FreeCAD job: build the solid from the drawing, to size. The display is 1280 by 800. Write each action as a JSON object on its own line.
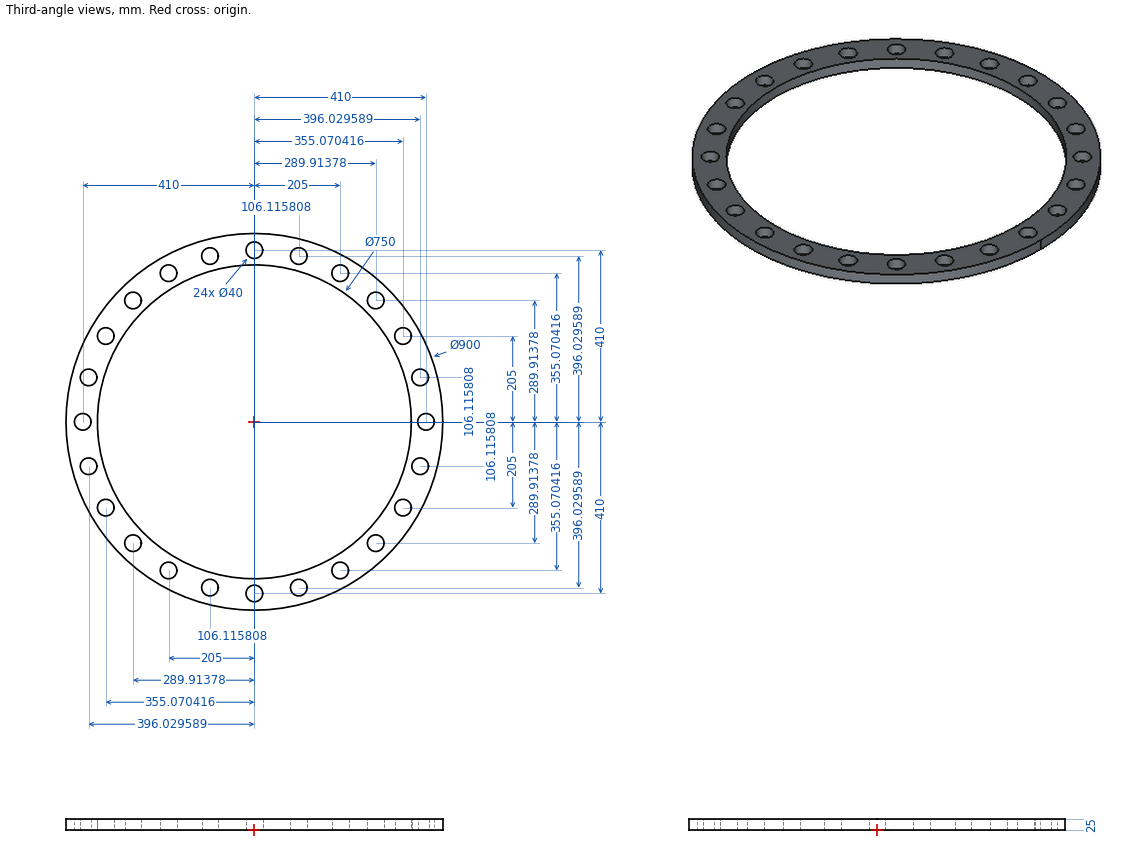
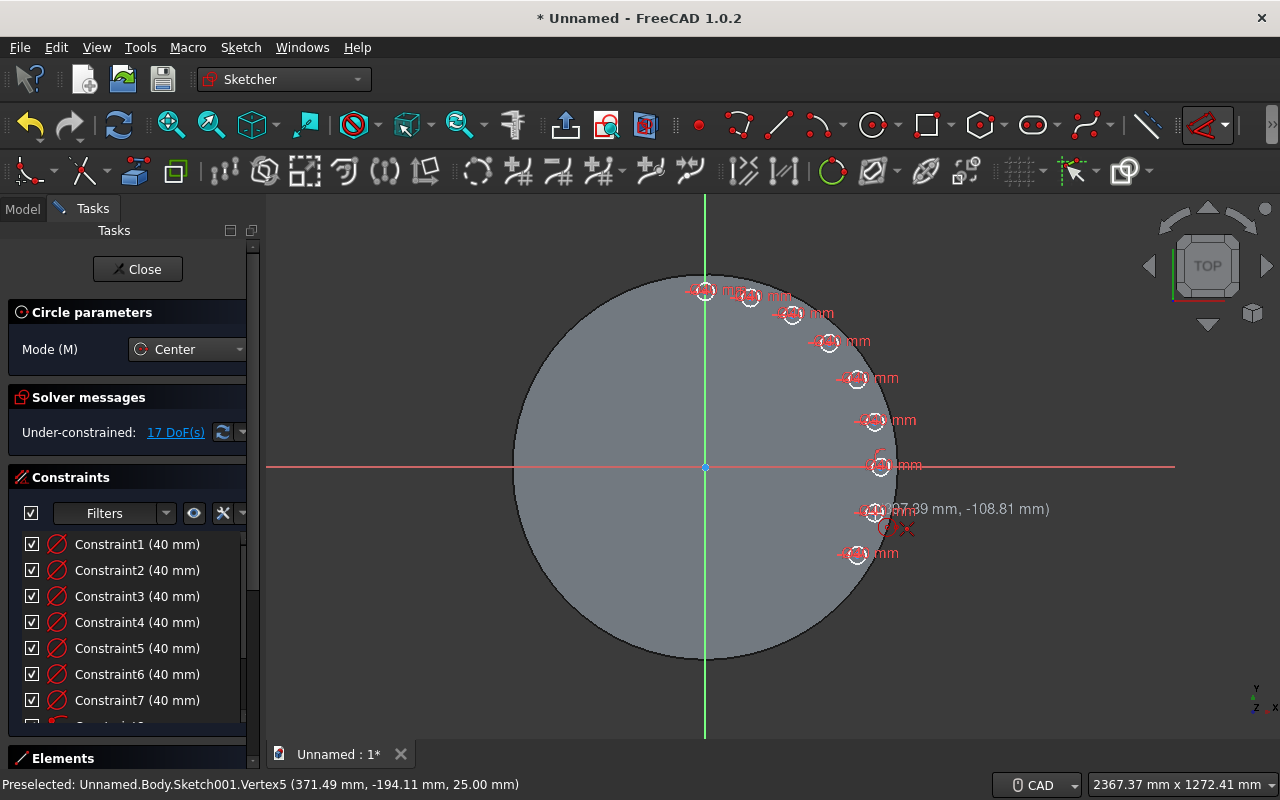
{"action": "scroll", "coordinate": [829, 591], "scroll_direction": "up", "scroll_amount": 5}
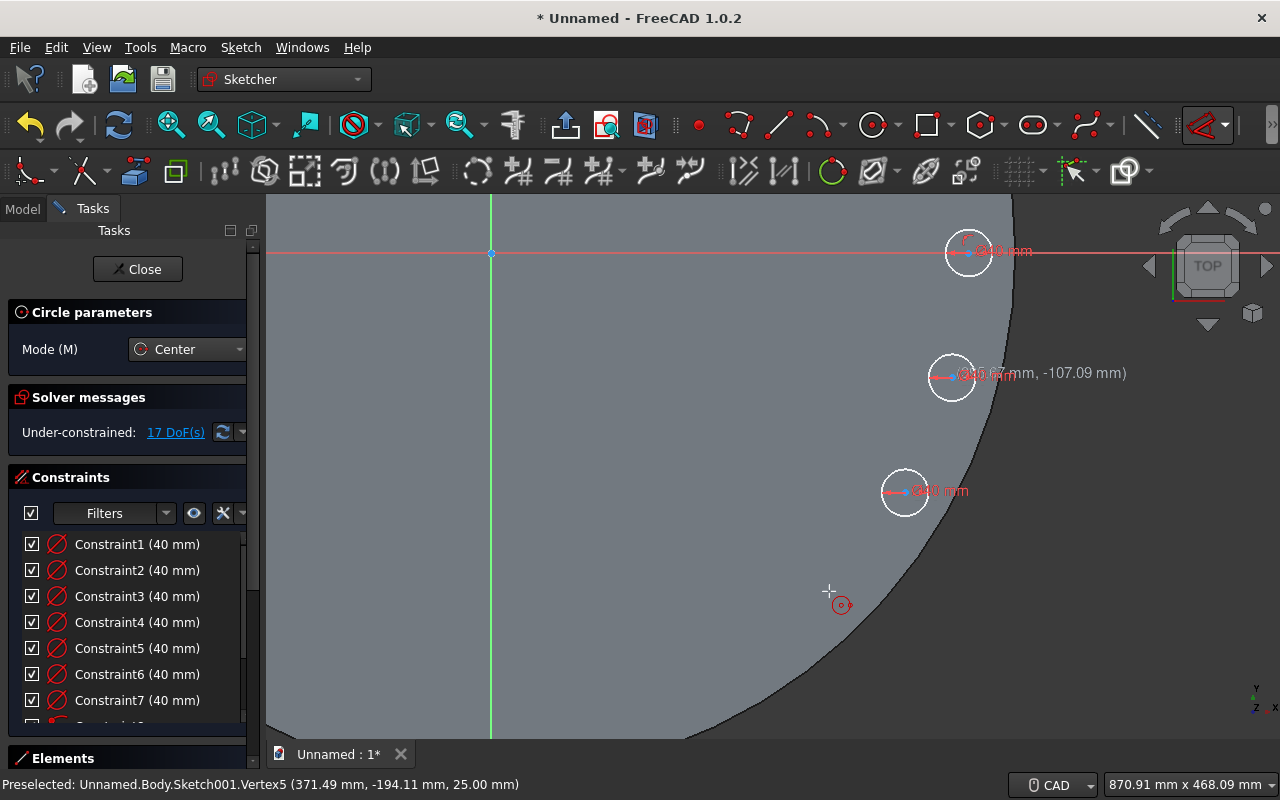
{"action": "left_click", "coordinate": [829, 591]}
{"action": "mouse_move", "coordinate": [845, 574]}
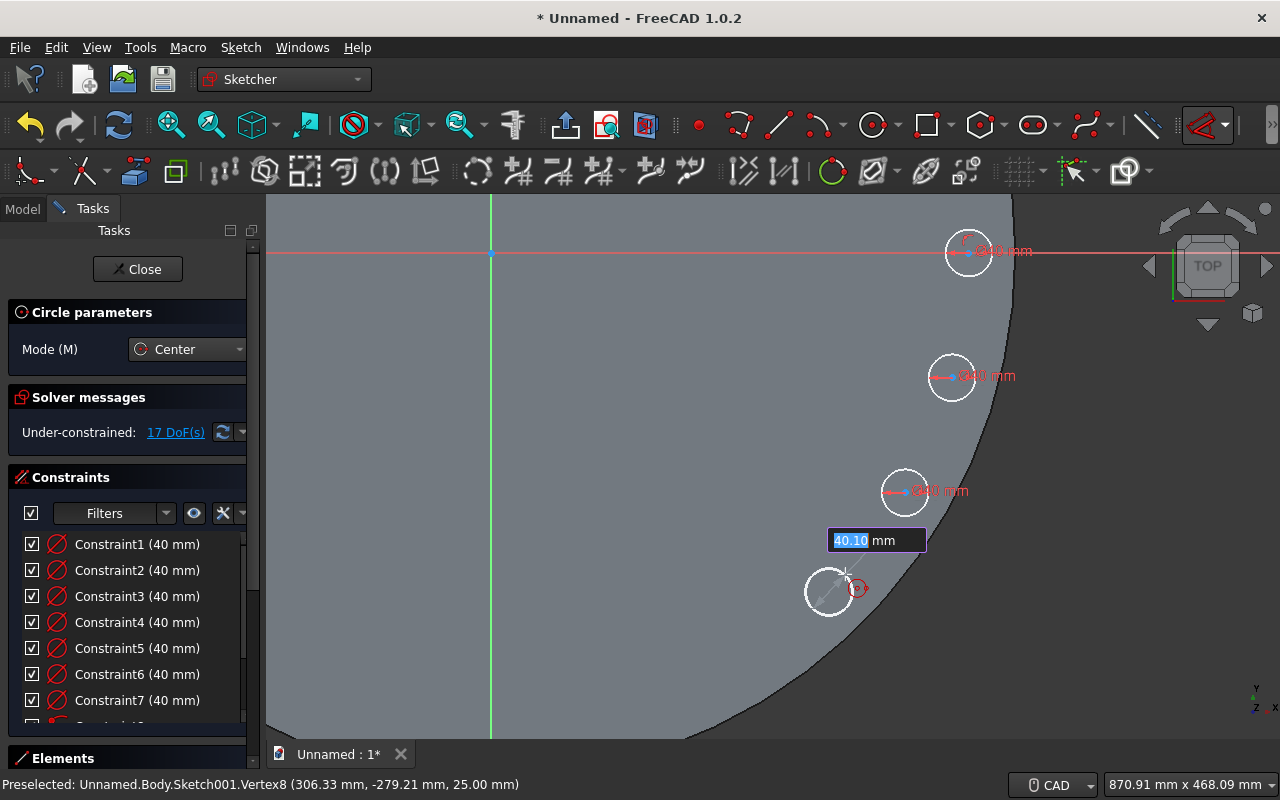
{"action": "type", "text": "40"}
{"action": "key", "text": "Return"}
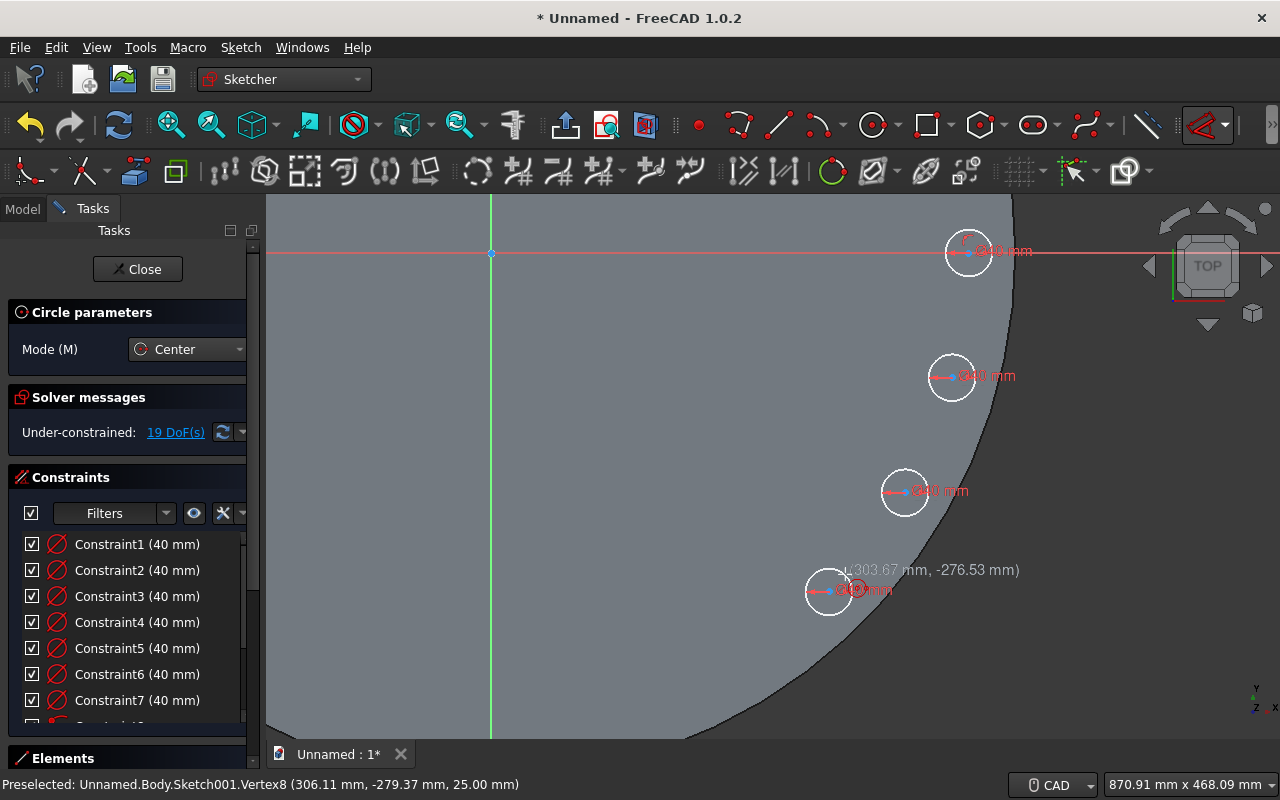
{"action": "left_click", "coordinate": [730, 666]}
{"action": "mouse_move", "coordinate": [747, 650]}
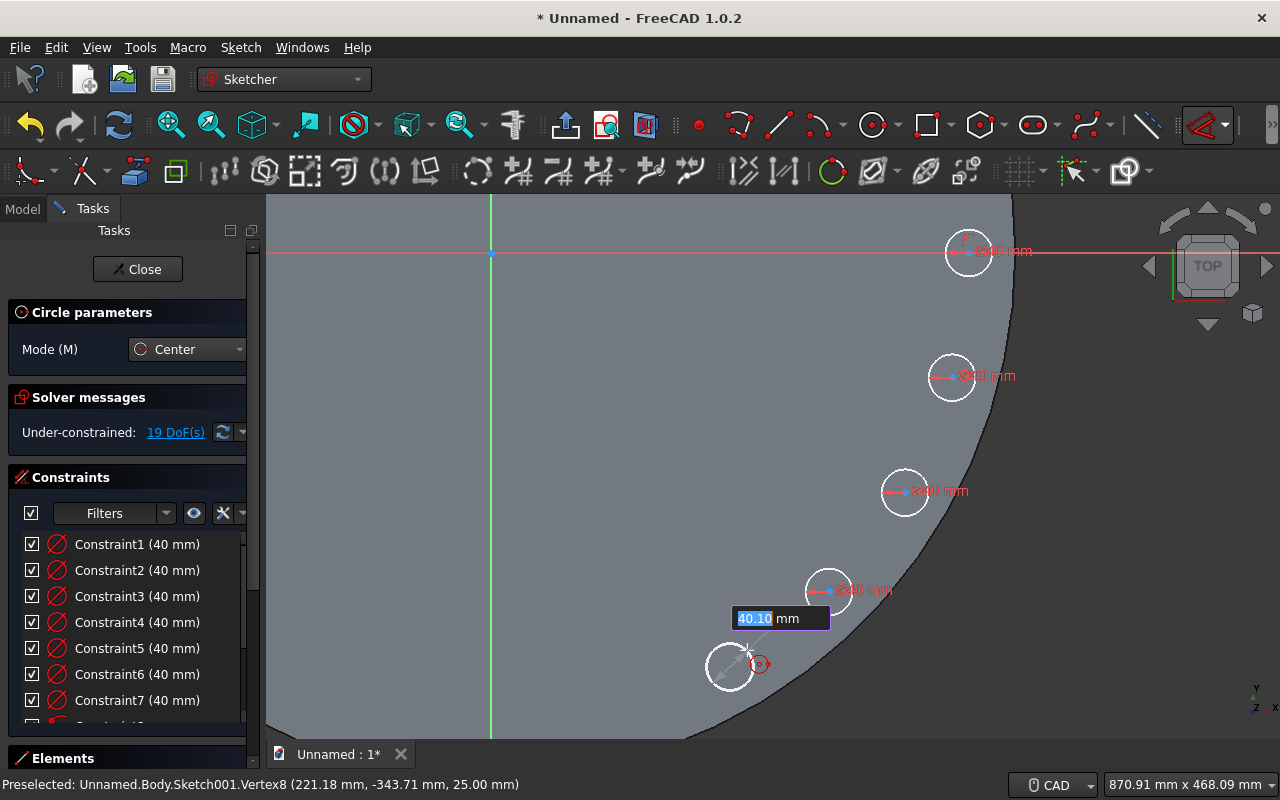
{"action": "type", "text": "40"}
{"action": "key", "text": "Return"}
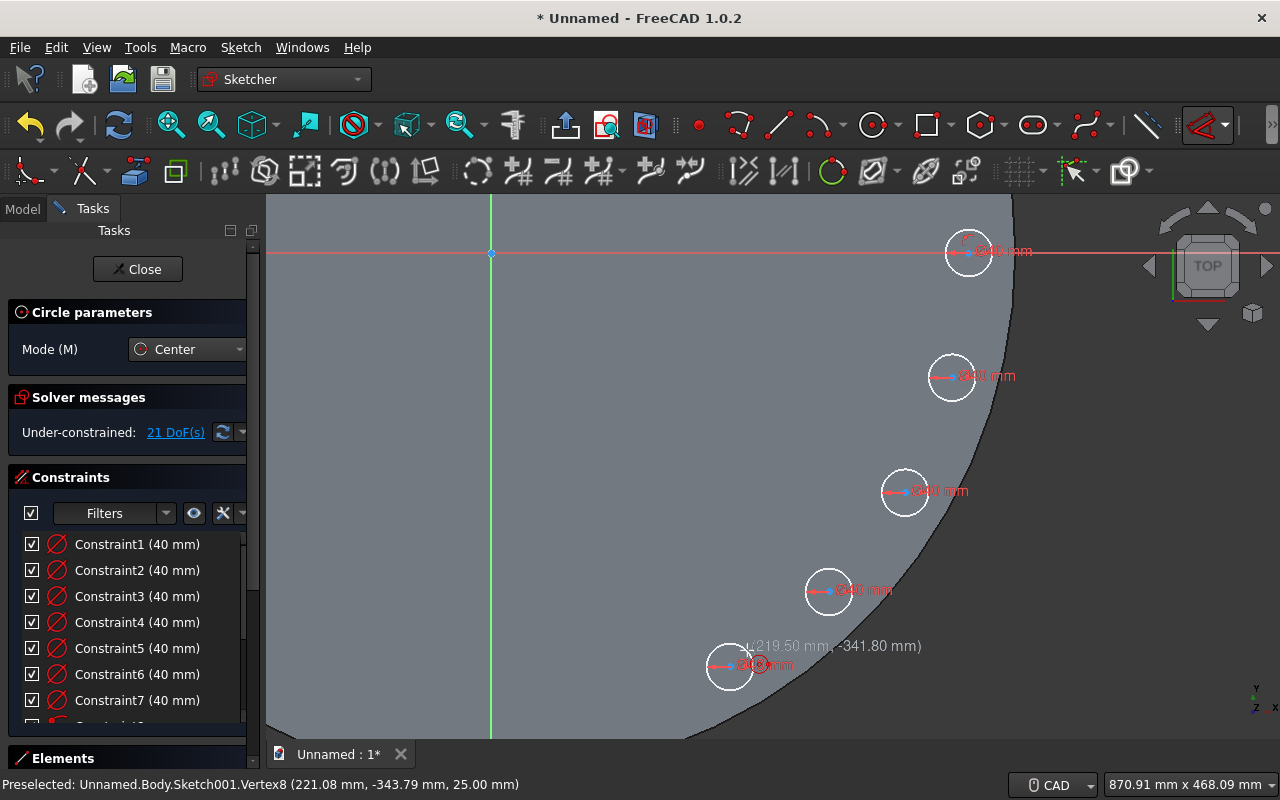
{"action": "scroll", "coordinate": [828, 591], "scroll_direction": "down", "scroll_amount": 5}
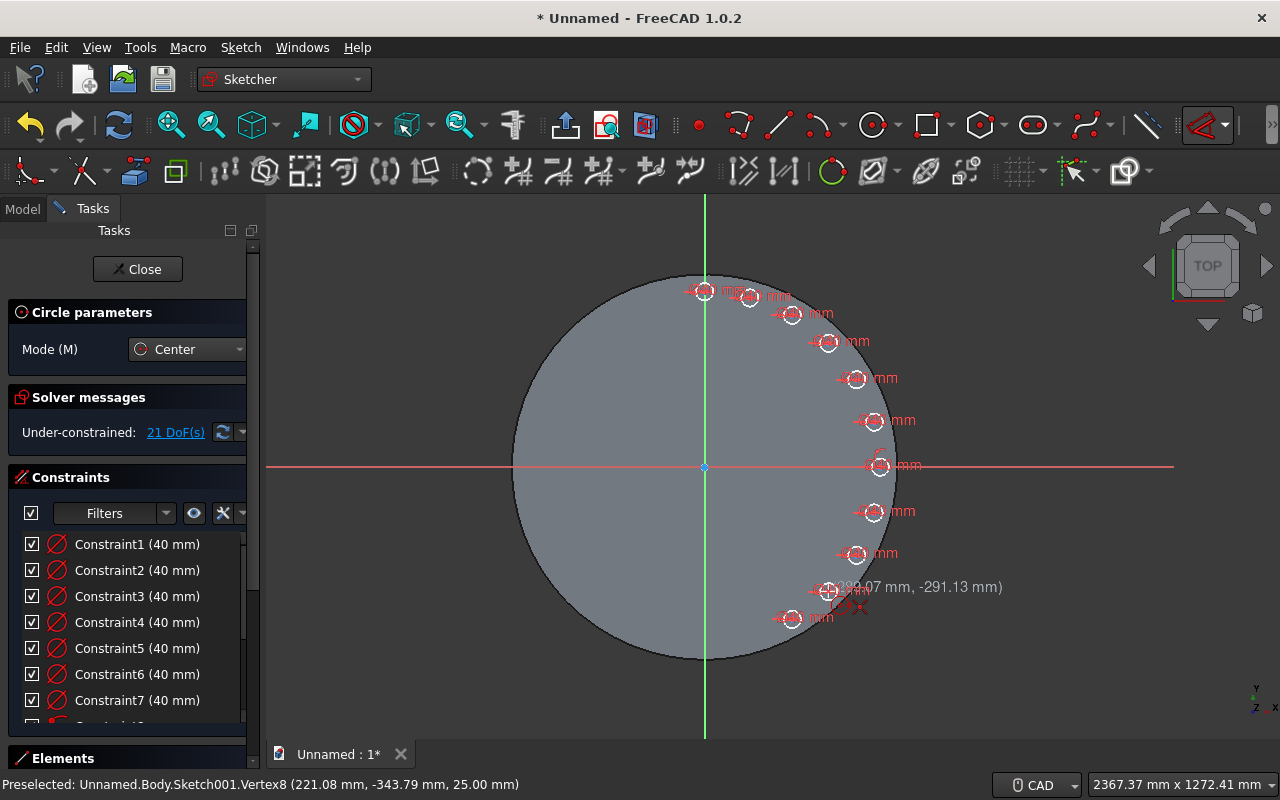
{"action": "scroll", "coordinate": [750, 637], "scroll_direction": "up", "scroll_amount": 5}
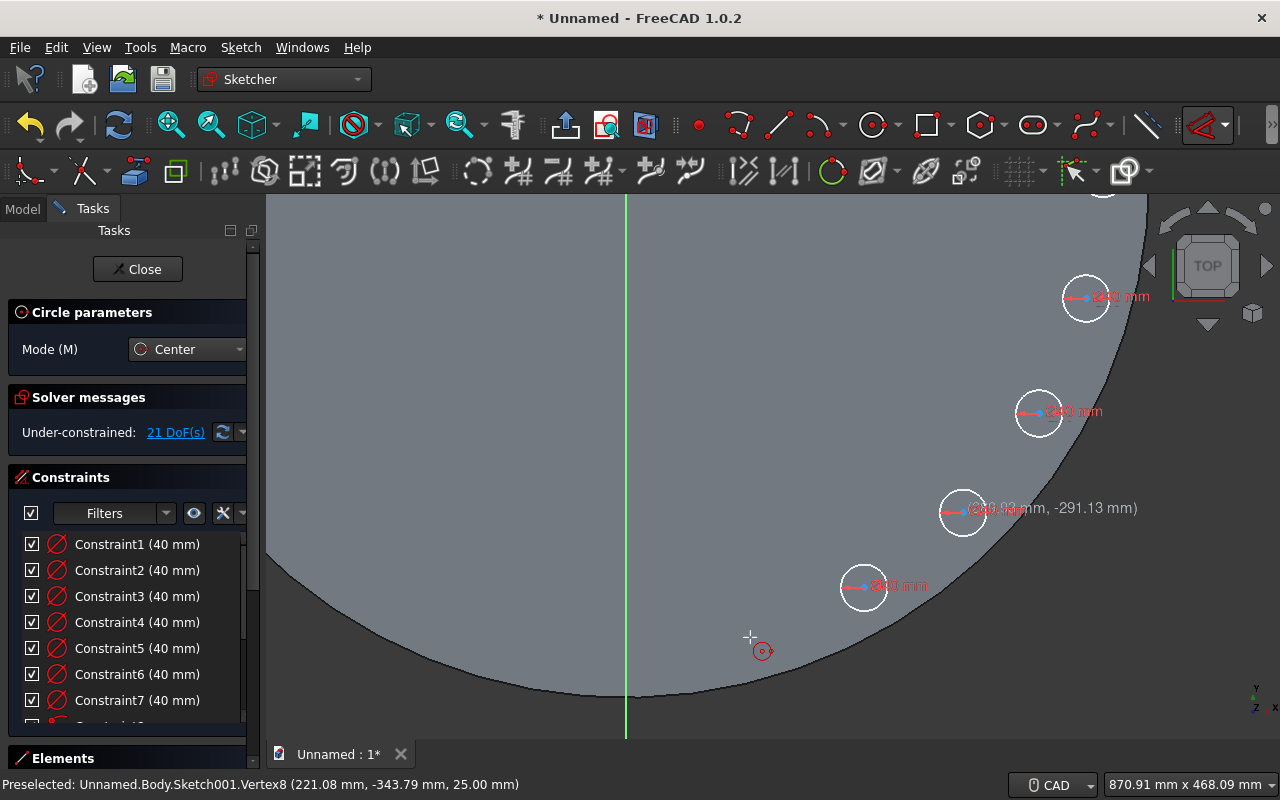
{"action": "left_click", "coordinate": [749, 635]}
{"action": "mouse_move", "coordinate": [766, 618]}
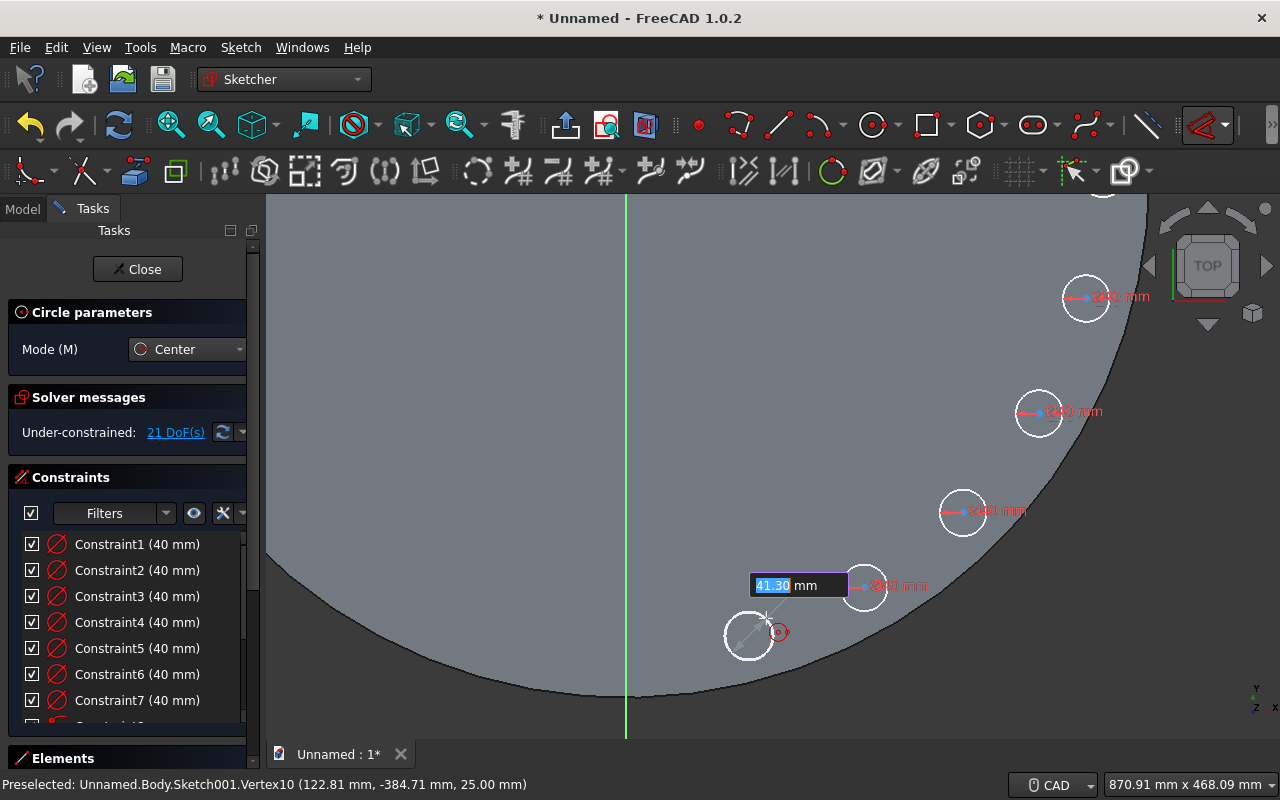
{"action": "type", "text": "40"}
{"action": "key", "text": "Return"}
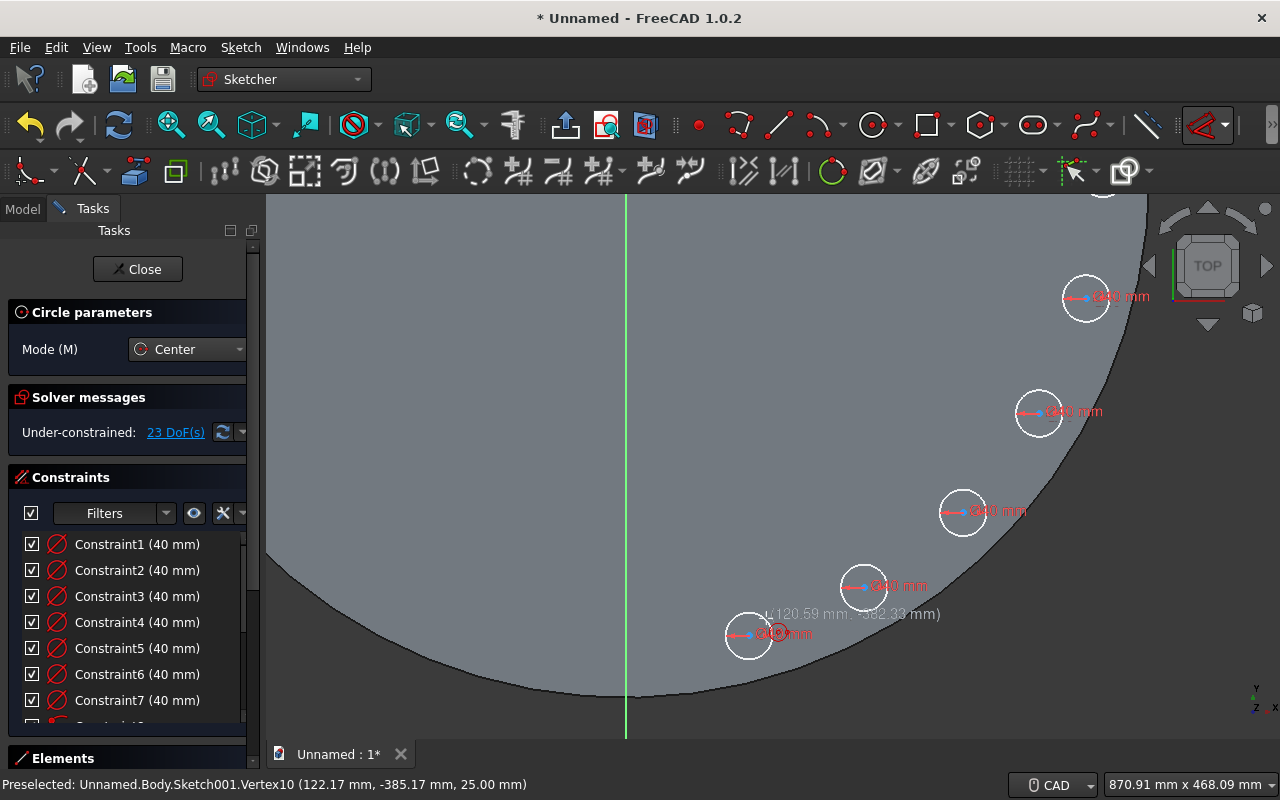
{"action": "left_click", "coordinate": [626, 651]}
{"action": "mouse_move", "coordinate": [642, 635]}